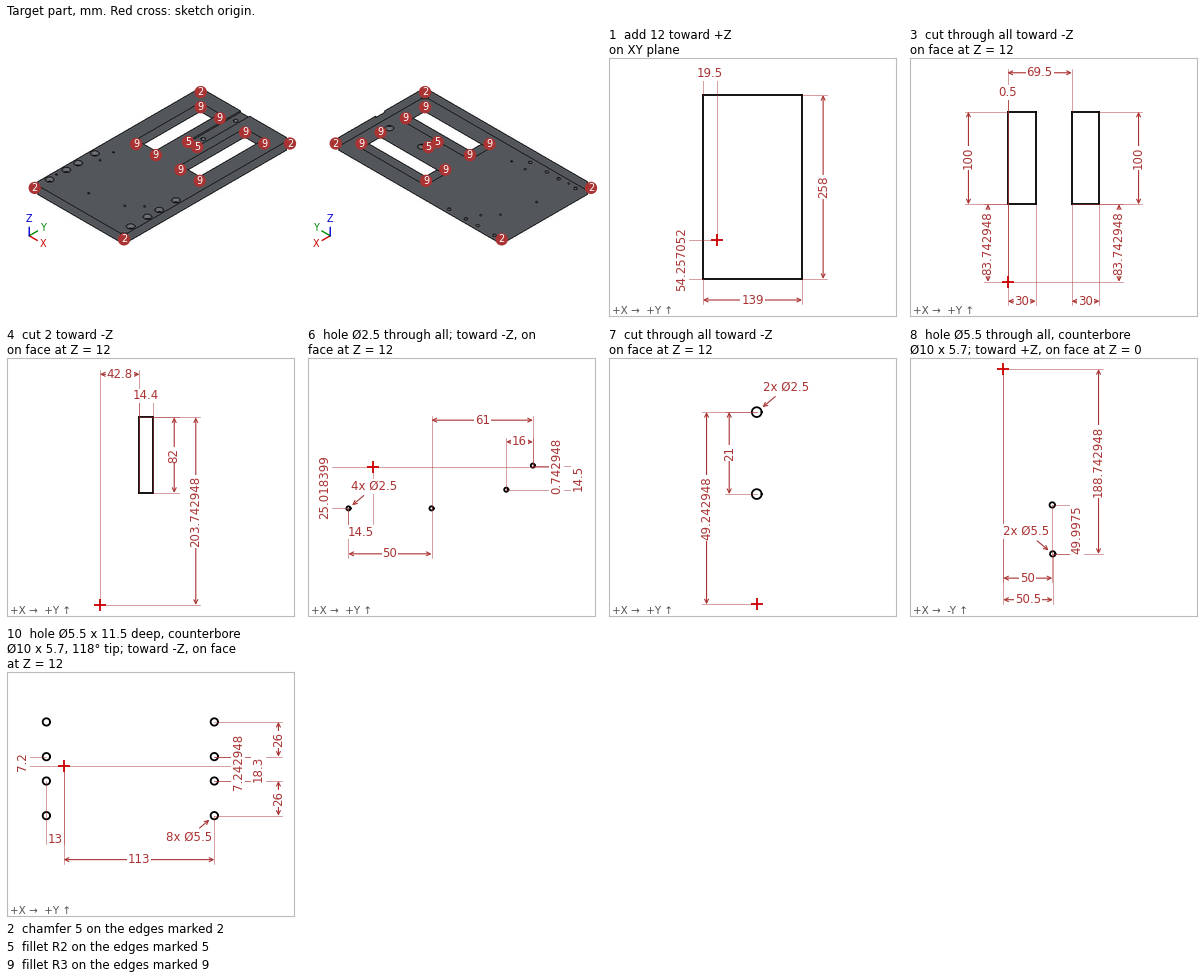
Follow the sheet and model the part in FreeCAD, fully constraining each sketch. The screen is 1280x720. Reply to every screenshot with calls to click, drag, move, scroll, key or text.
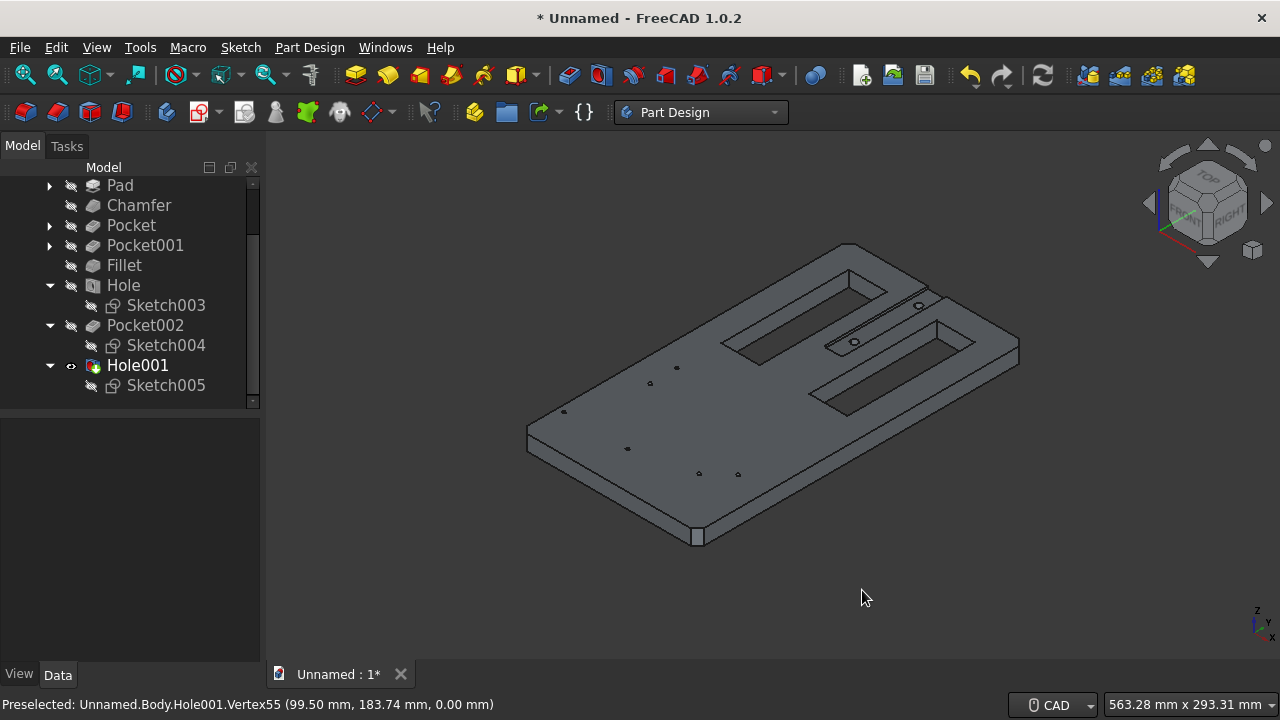
scroll(975, 350, up, 4)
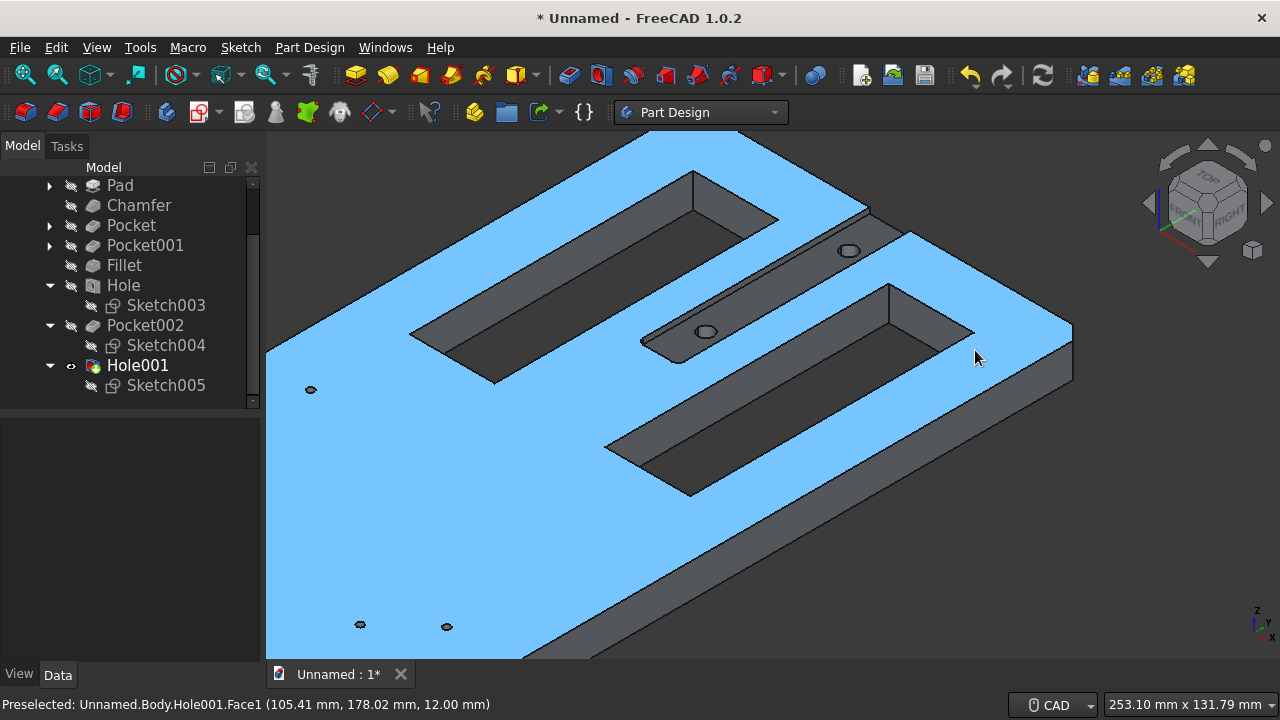
key(v)
key(f)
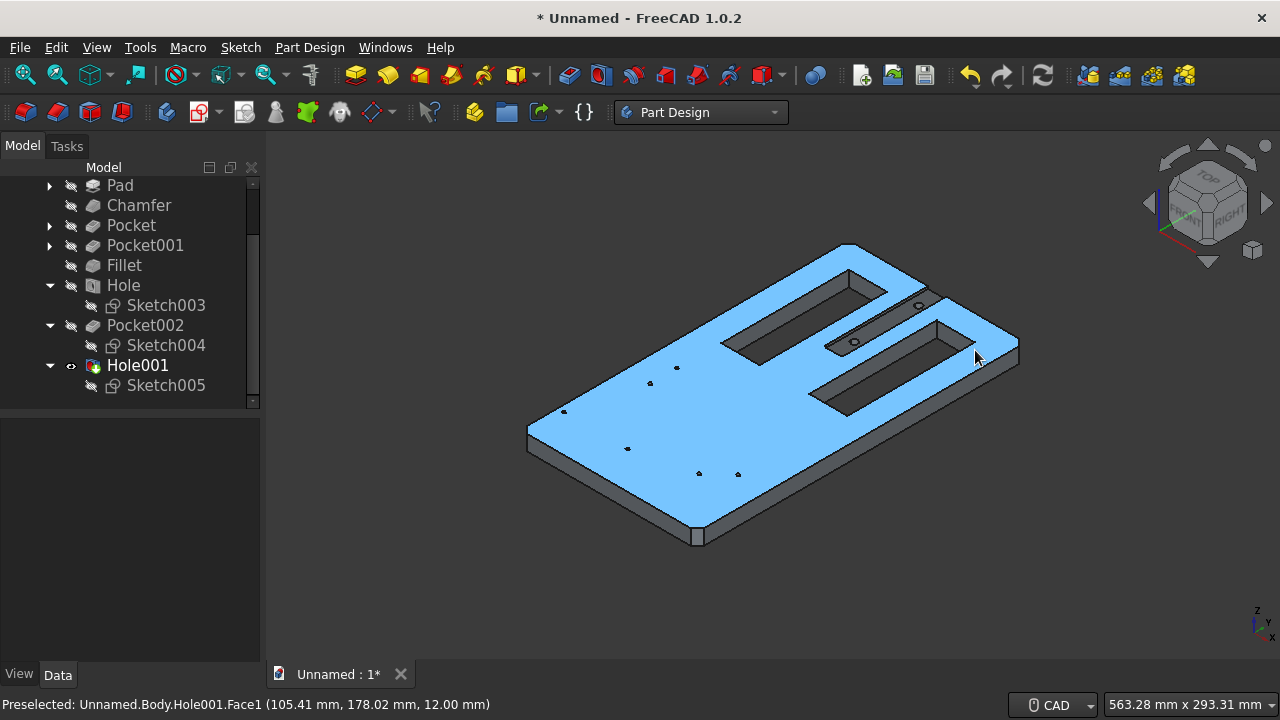
key(2)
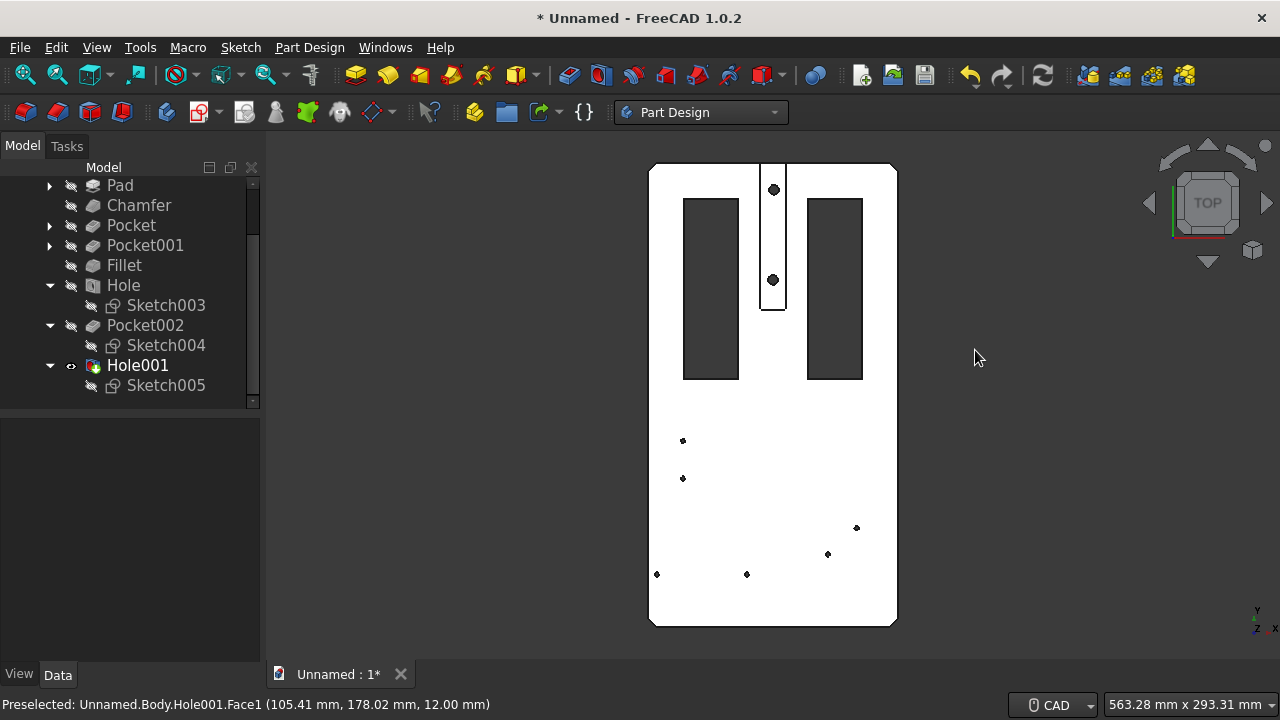
scroll(862, 198, up, 4)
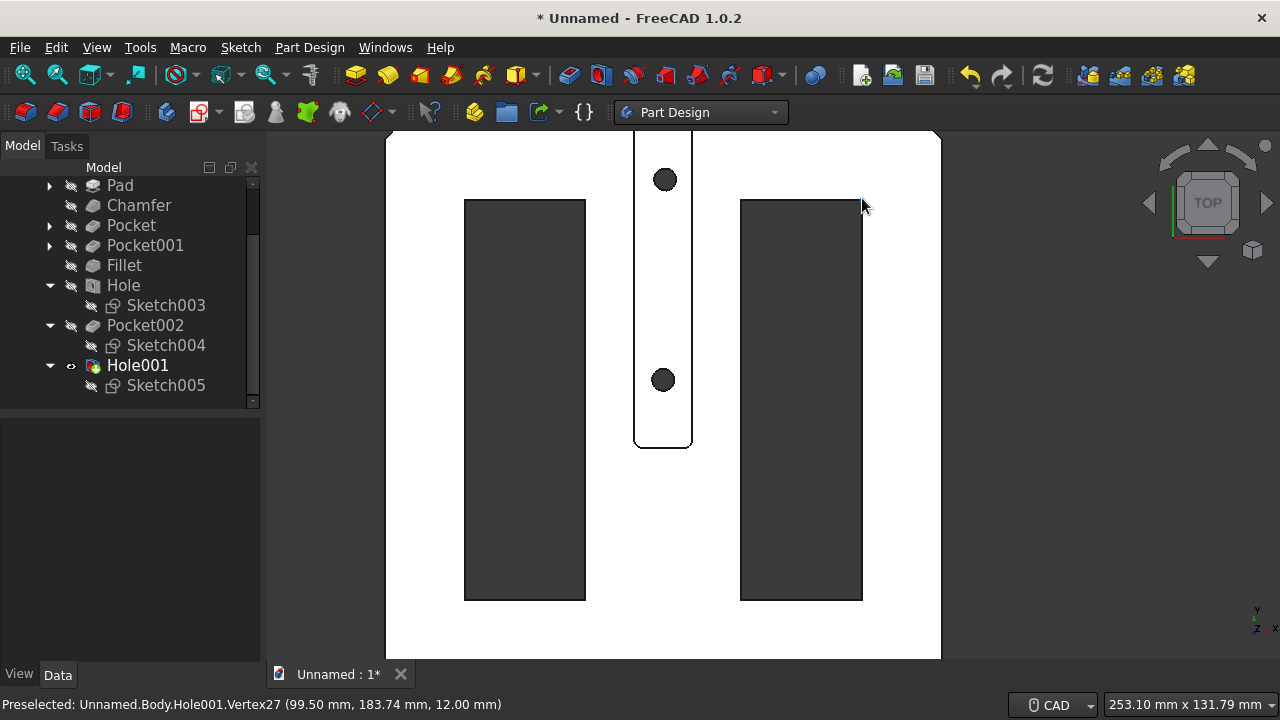
key(v)
key(f)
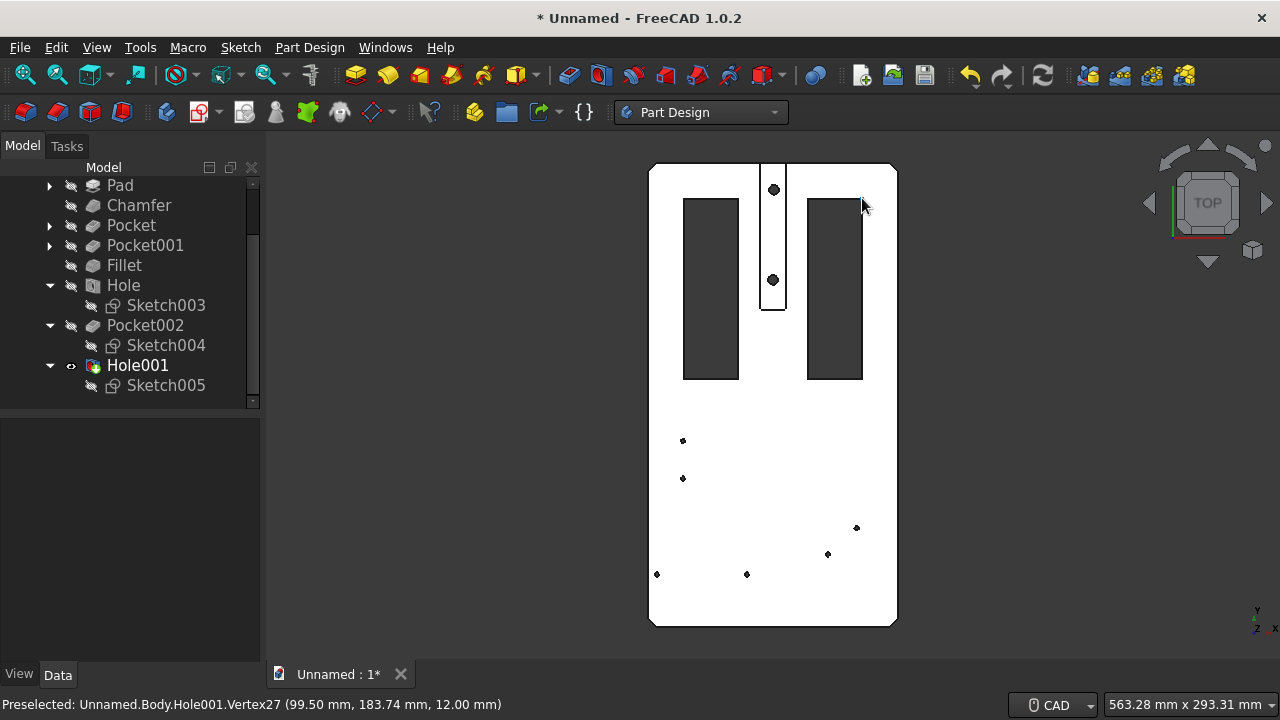
key(1)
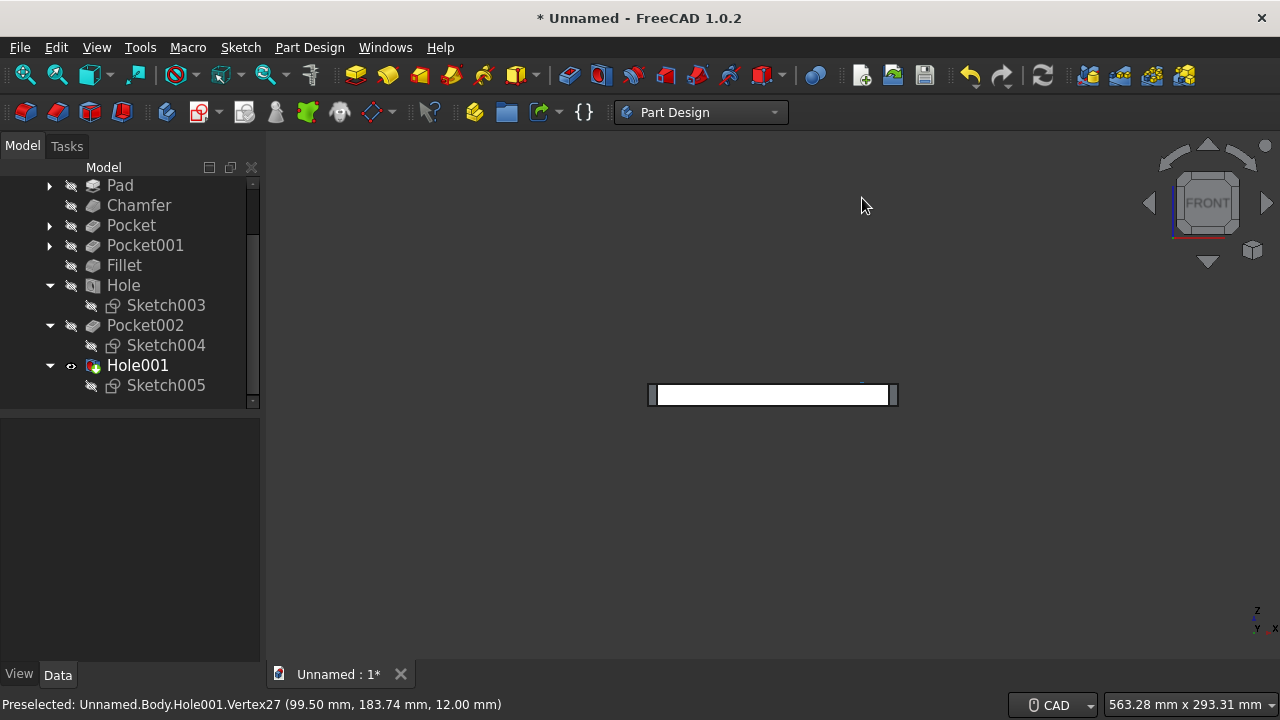
key(v)
key(f)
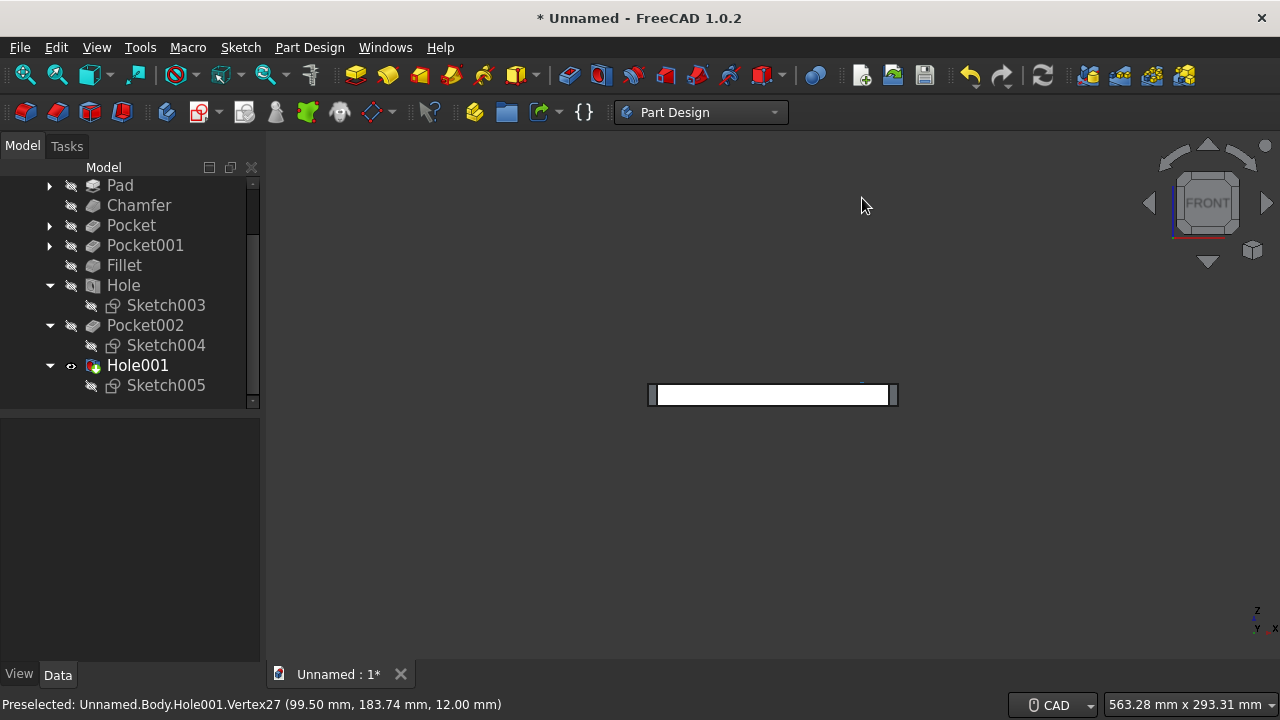
scroll(862, 394, up, 4)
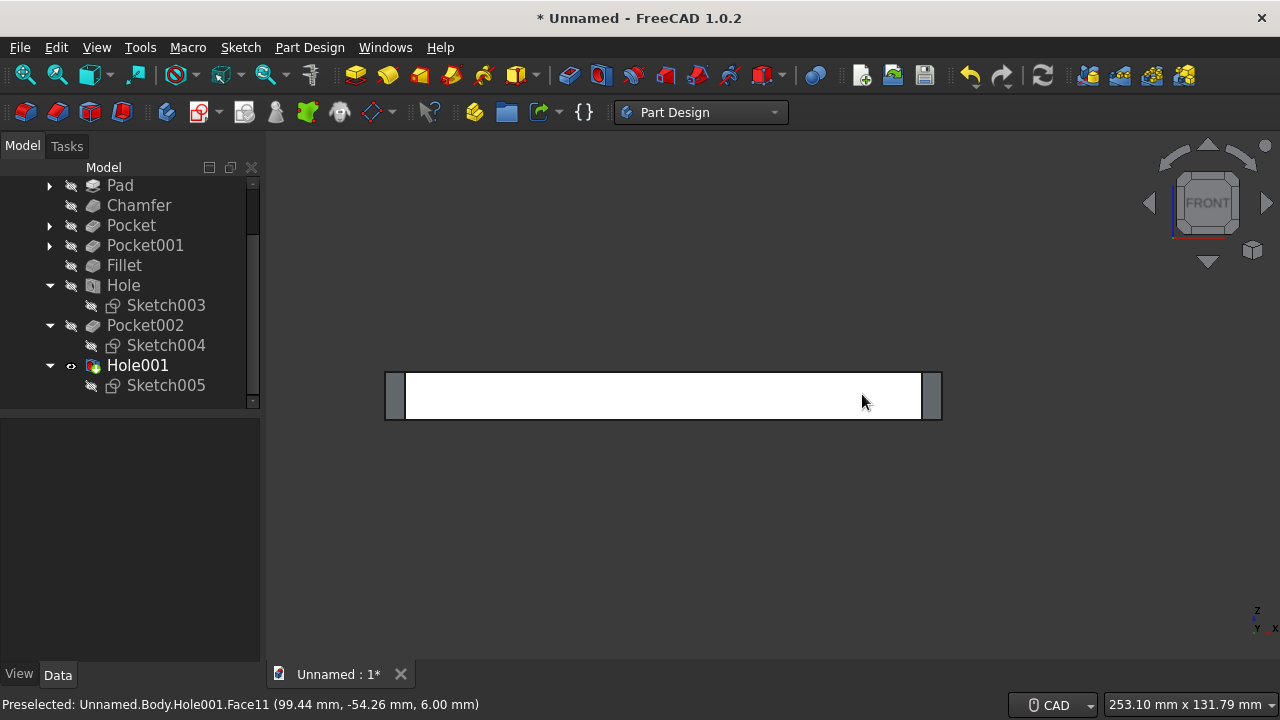
key(v)
key(f)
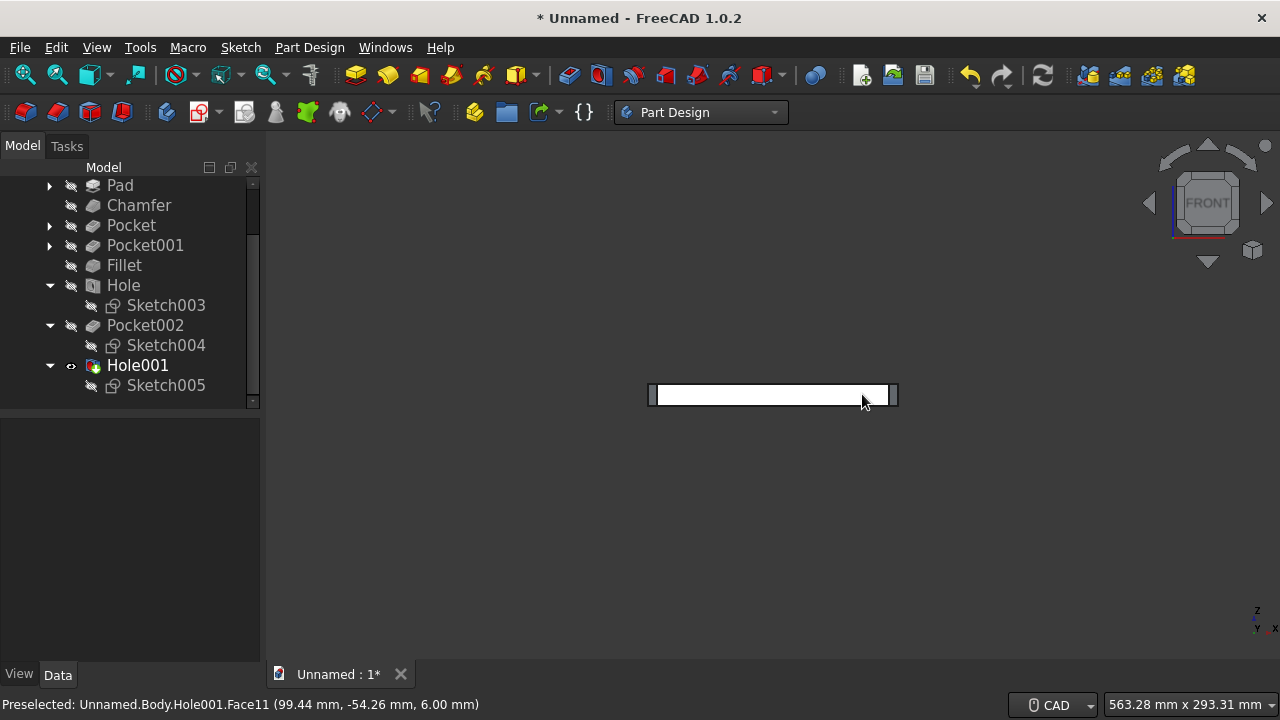
key(3)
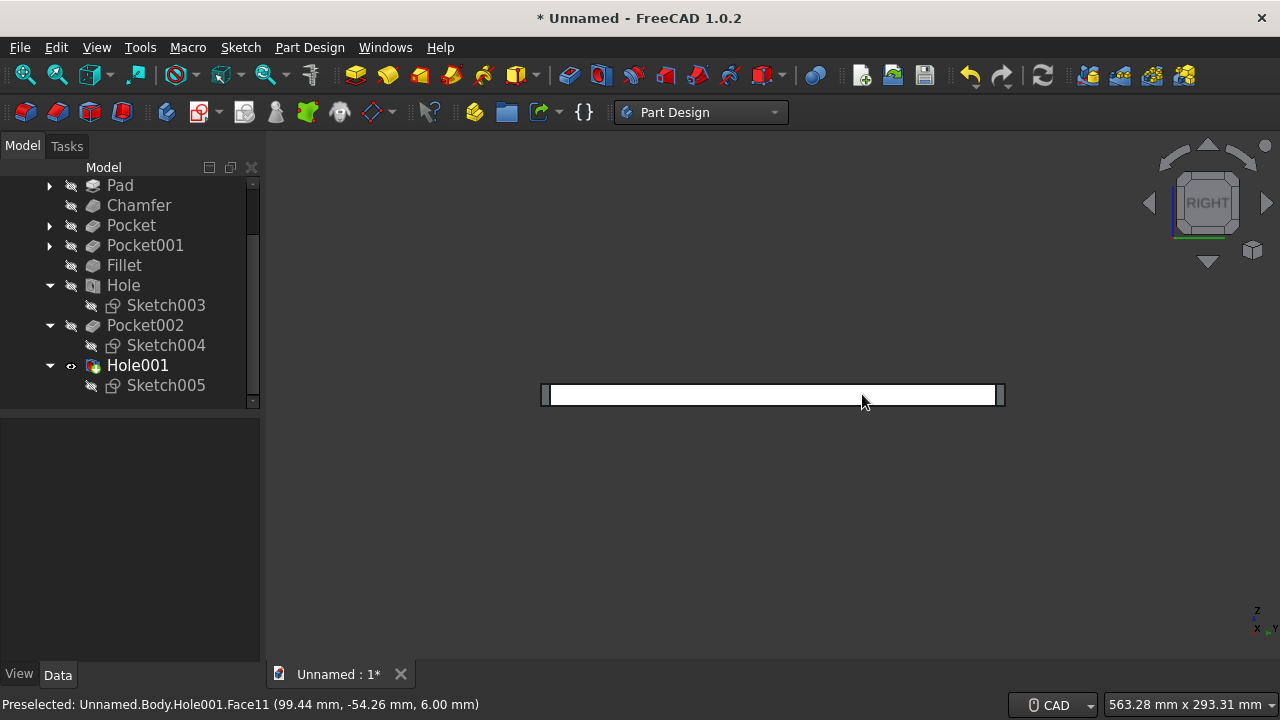
scroll(969, 394, up, 4)